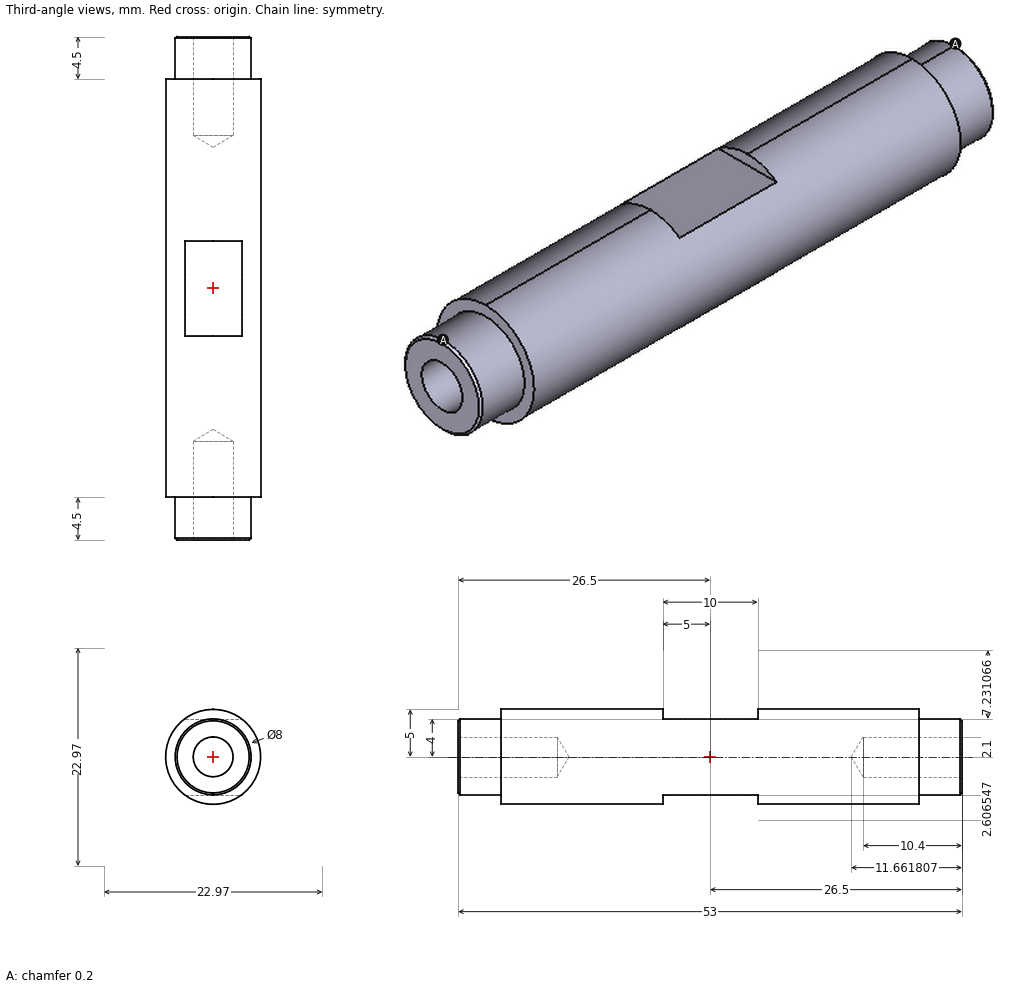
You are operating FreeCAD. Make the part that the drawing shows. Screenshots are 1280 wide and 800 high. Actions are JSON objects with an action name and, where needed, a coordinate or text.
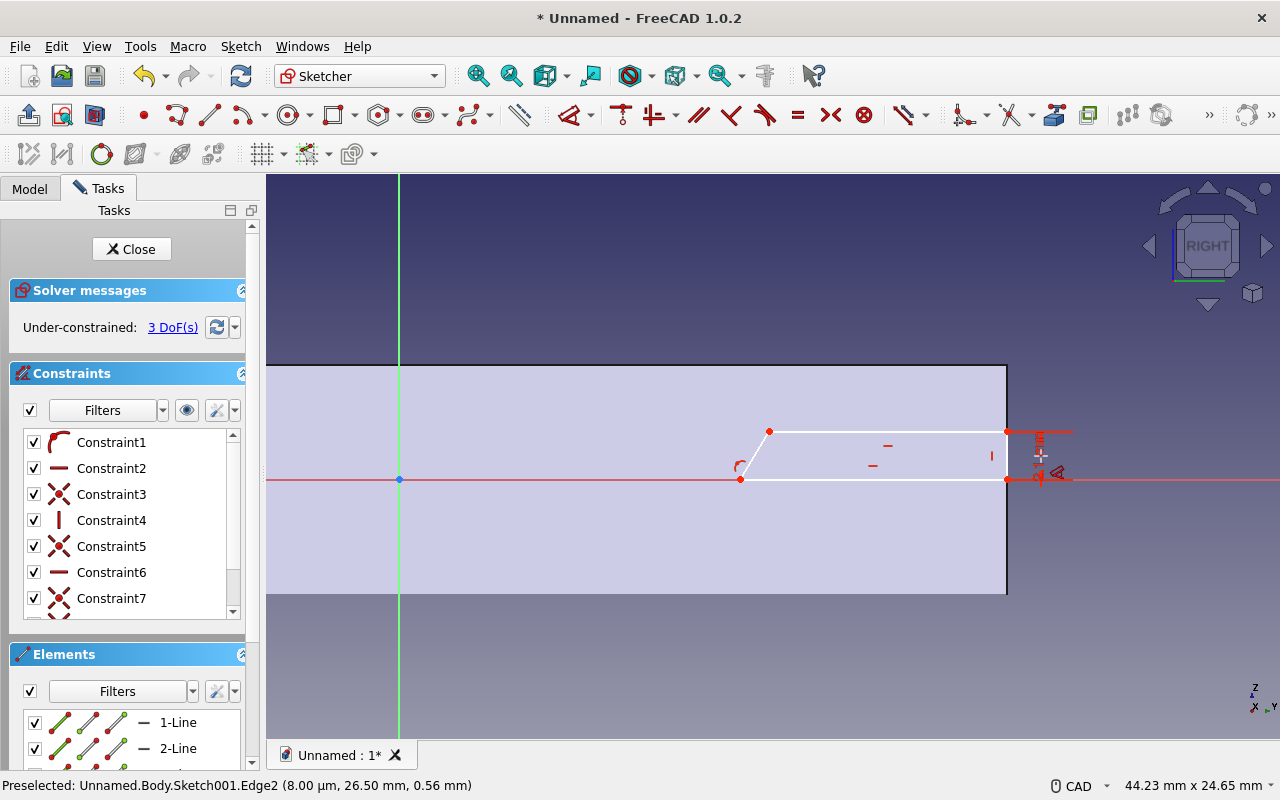
{"action": "left_click", "coordinate": [936, 432]}
{"action": "left_click", "coordinate": [888, 398]}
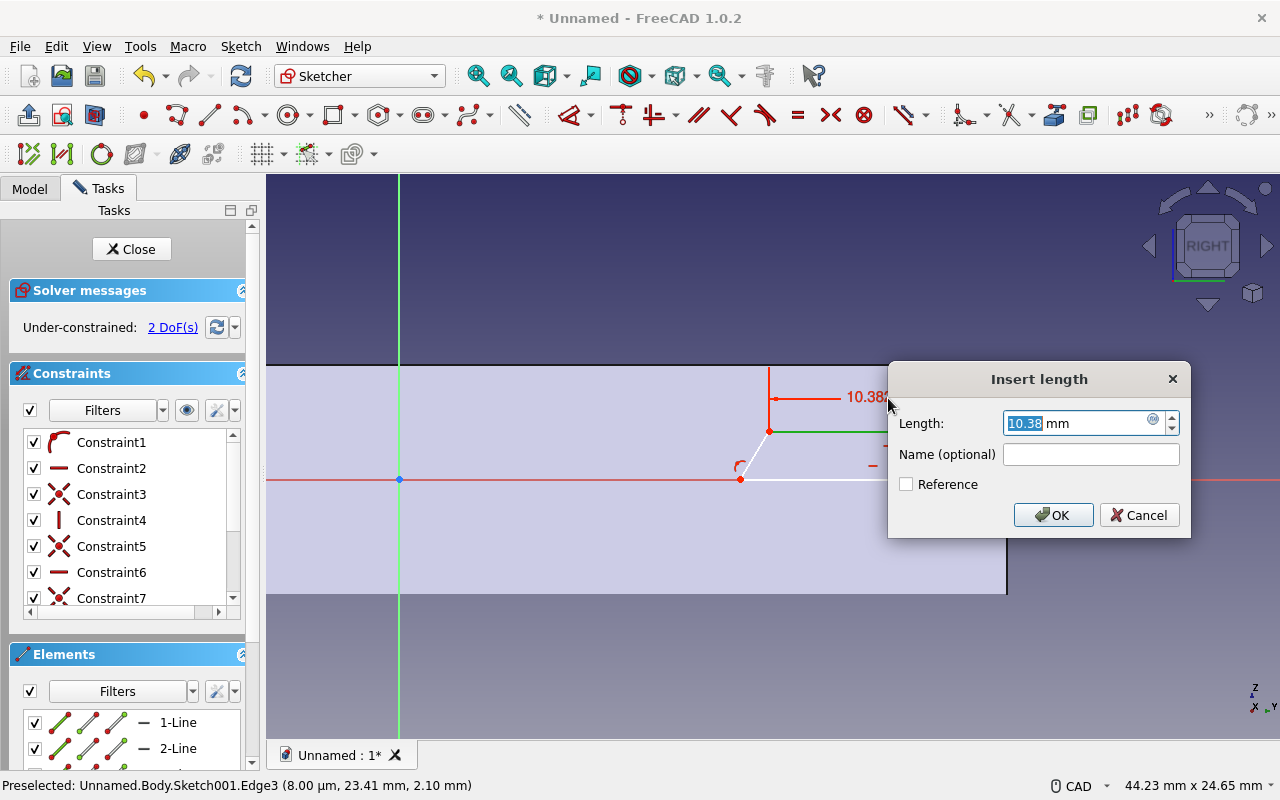
{"action": "type", "text": "10.4"}
{"action": "key", "text": "Return"}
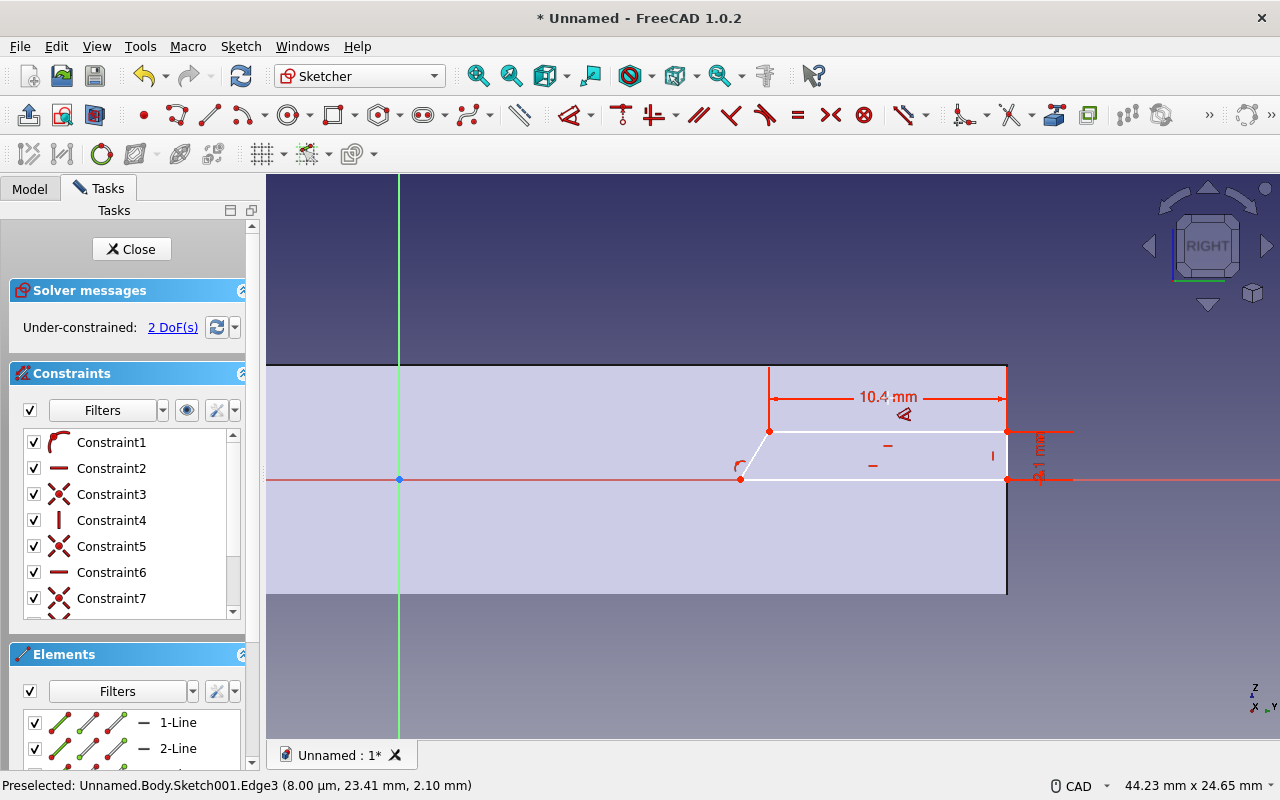
{"action": "left_click", "coordinate": [1007, 480]}
{"action": "left_click", "coordinate": [703, 514]}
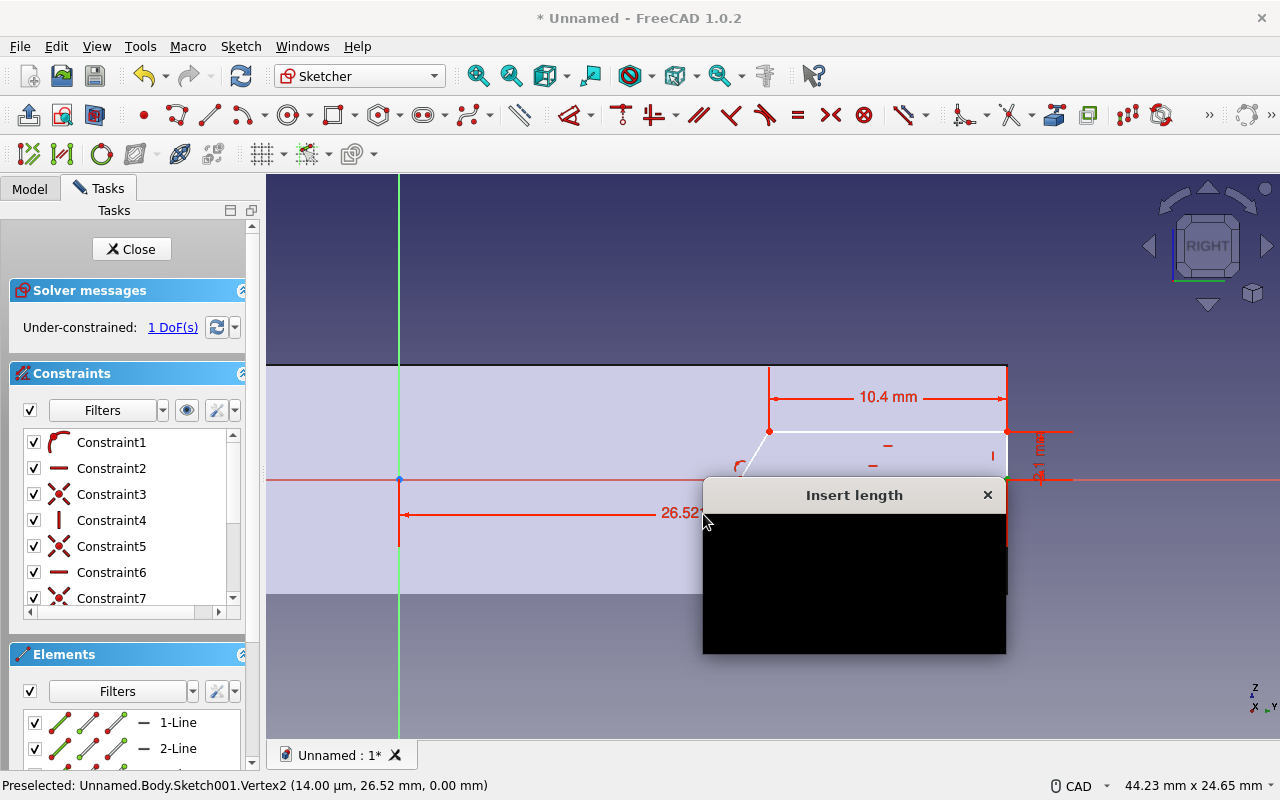
{"action": "type", "text": "26.5"}
{"action": "key", "text": "Return"}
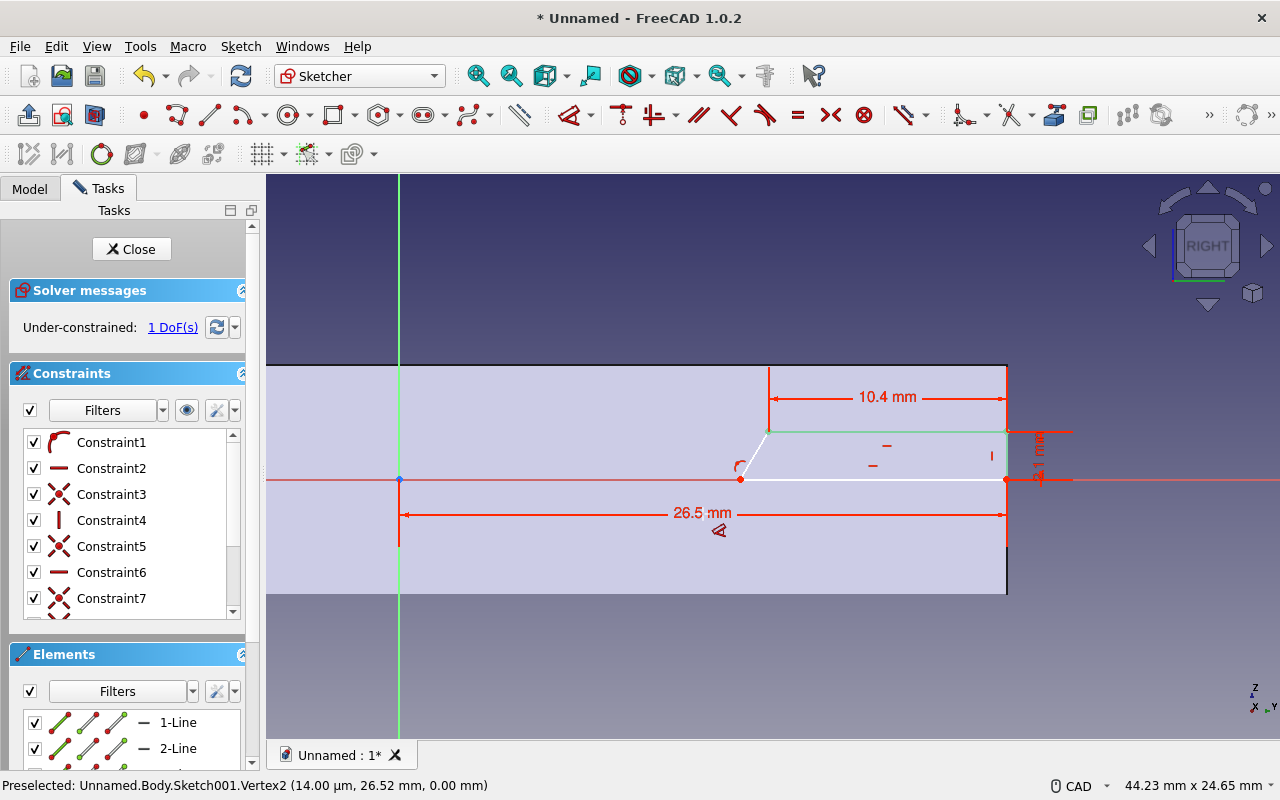
{"action": "left_click", "coordinate": [820, 480]}
{"action": "left_click", "coordinate": [873, 514]}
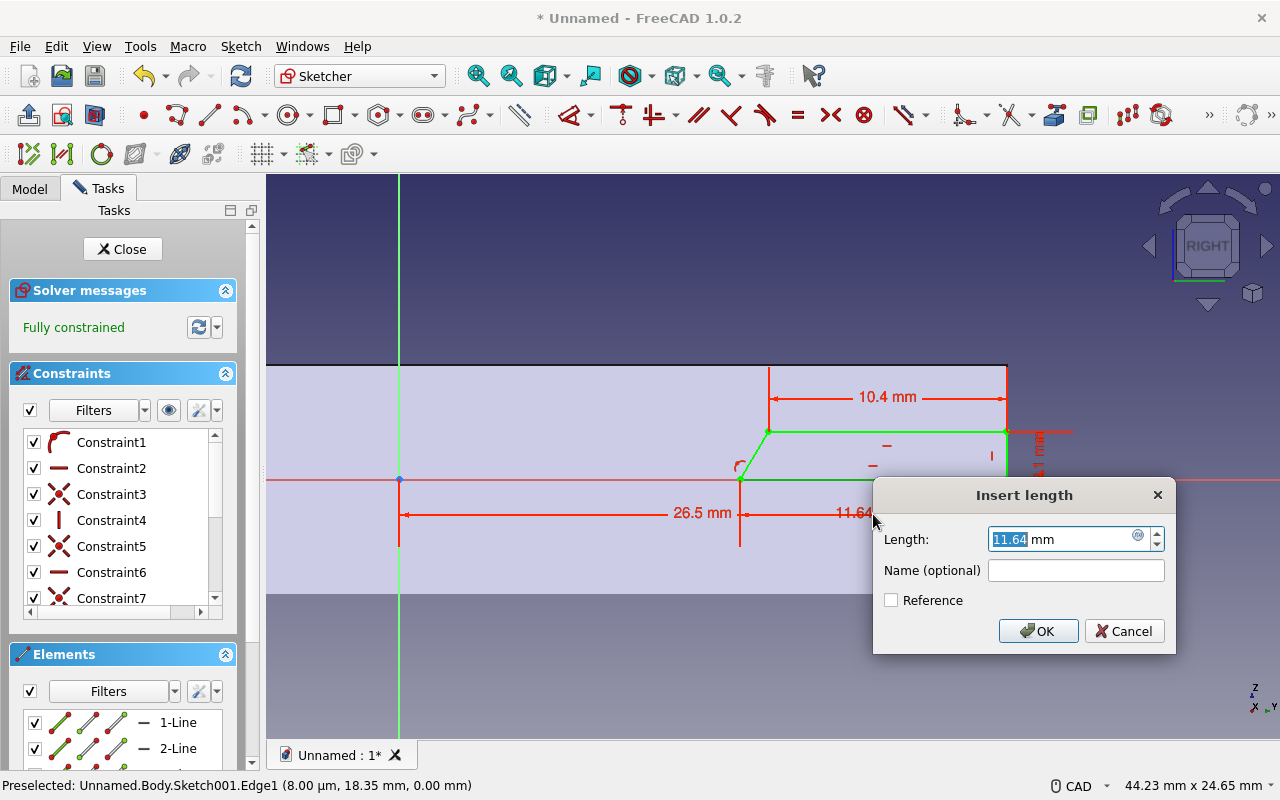
{"action": "type", "text": "11.661807"}
{"action": "key", "text": "Return"}
{"action": "key", "text": "Escape"}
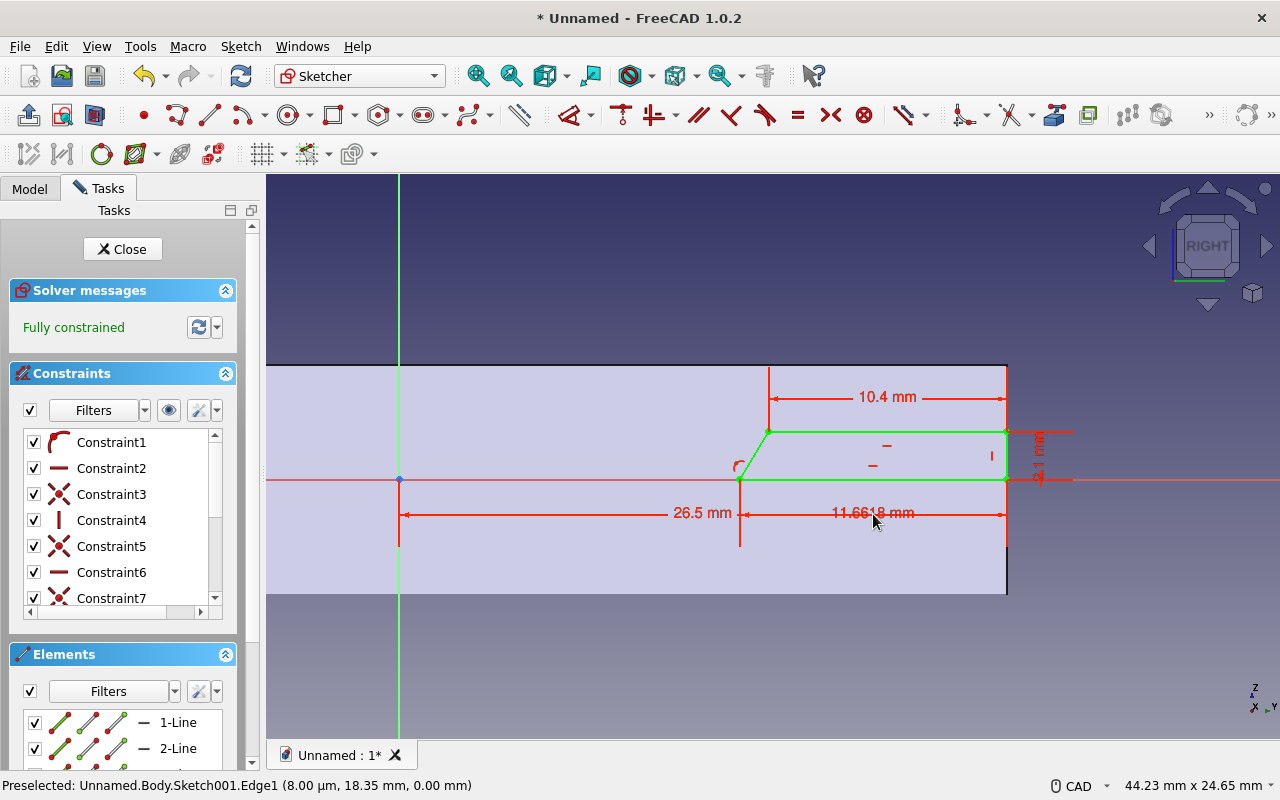
{"action": "left_click", "coordinate": [123, 249]}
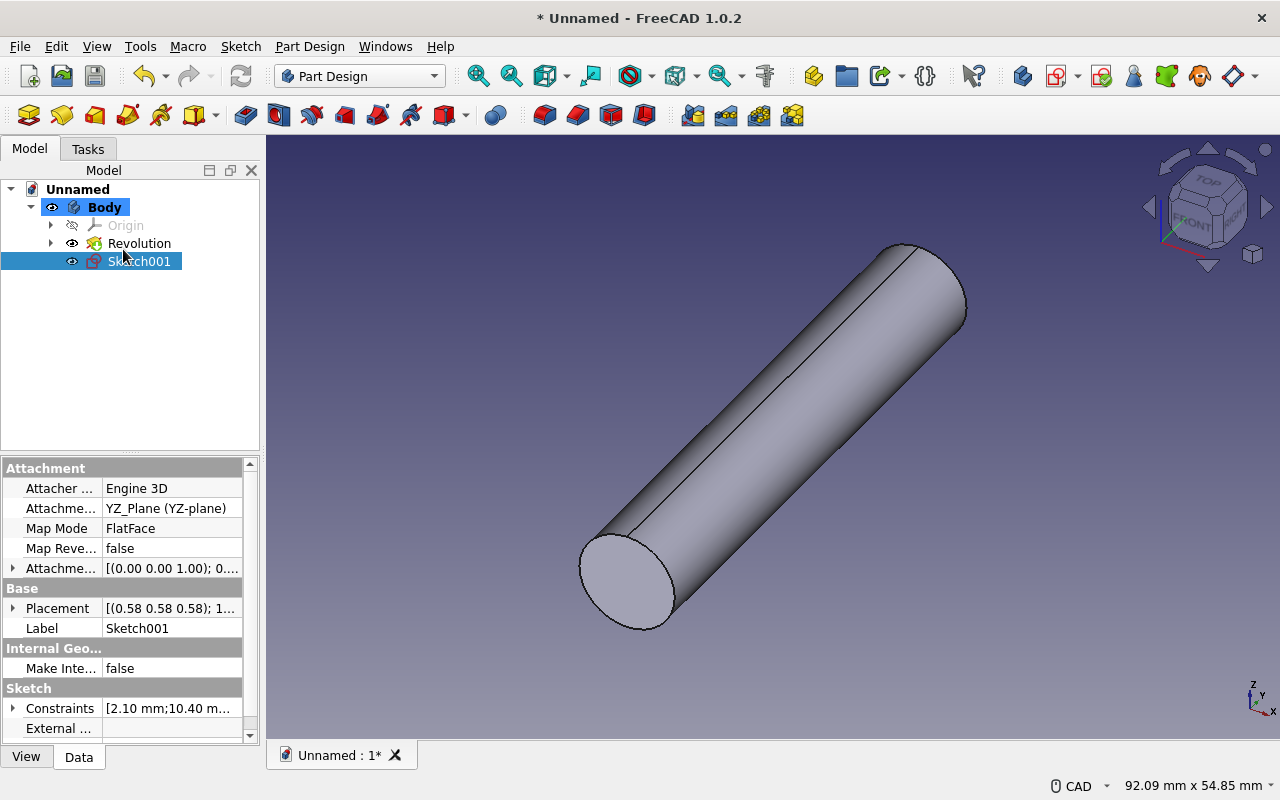
{"action": "left_click", "coordinate": [312, 116]}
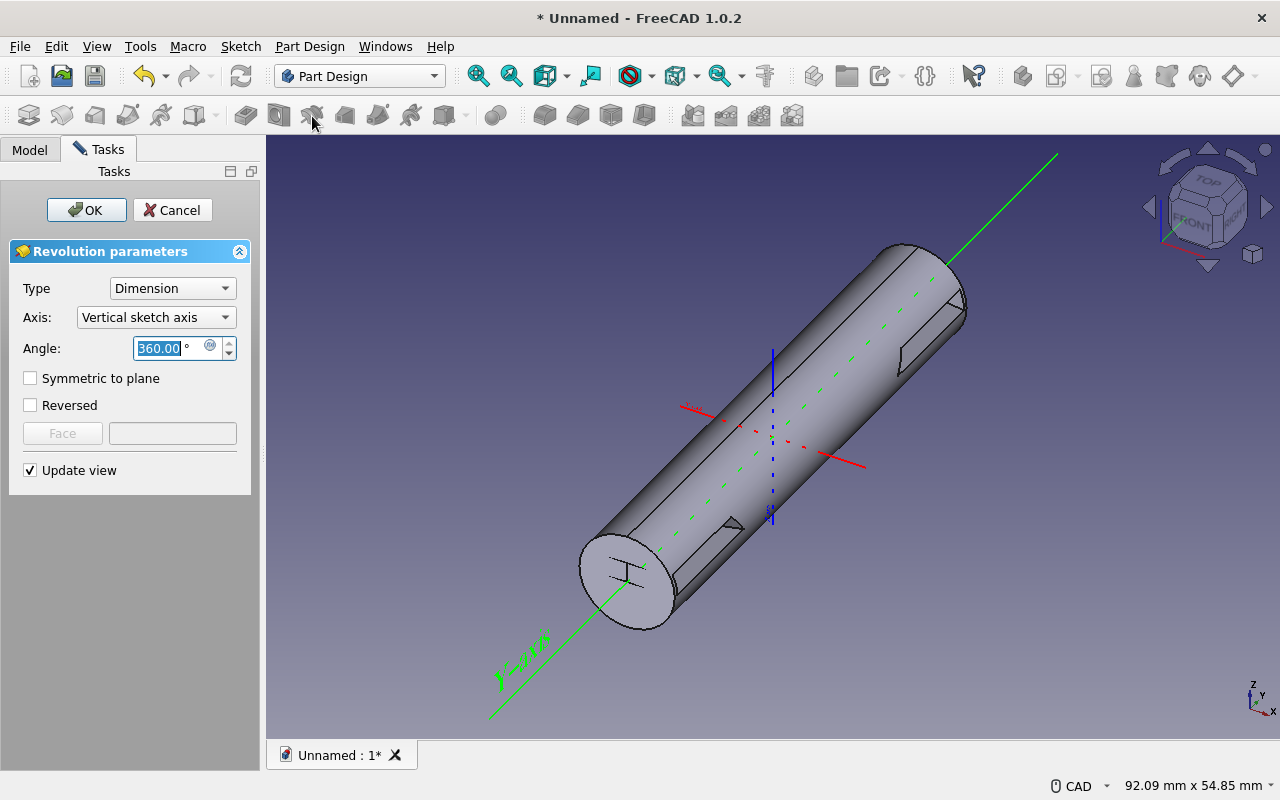
{"action": "left_click", "coordinate": [157, 318]}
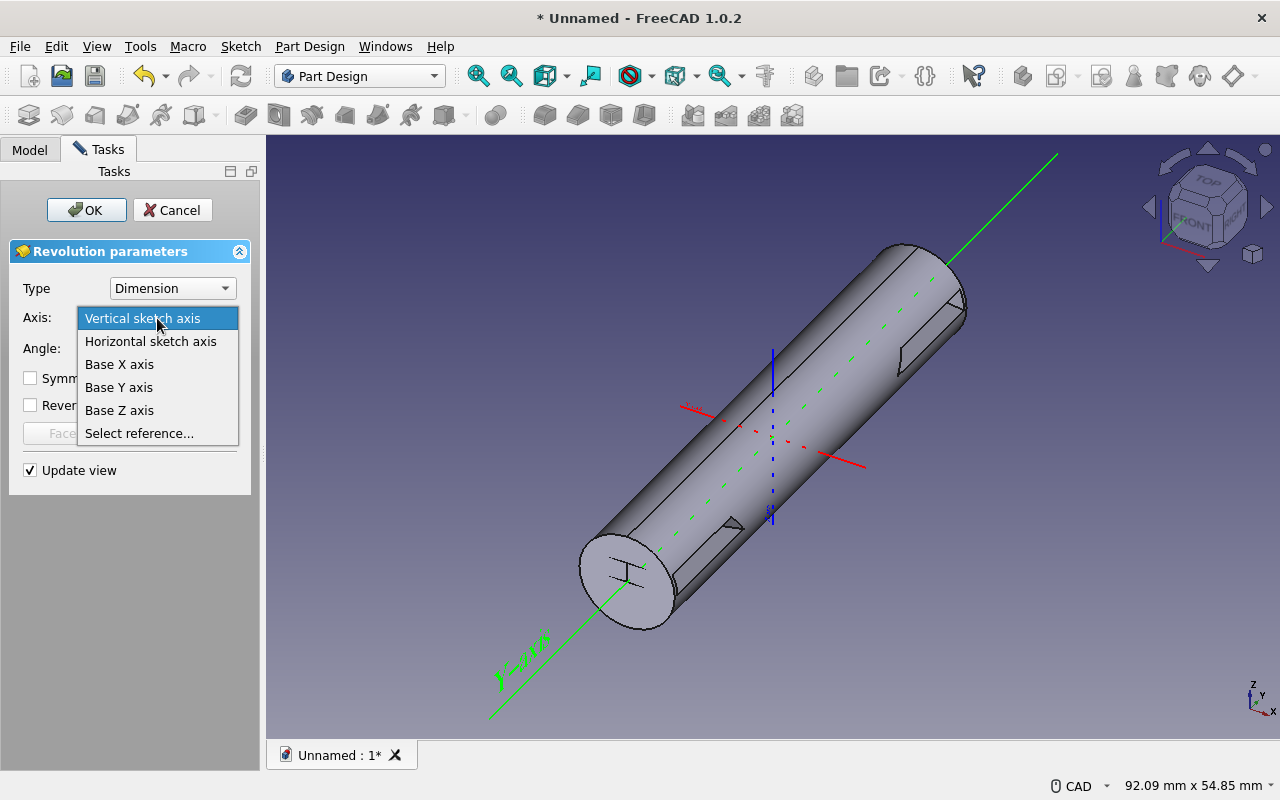
{"action": "left_click", "coordinate": [156, 342]}